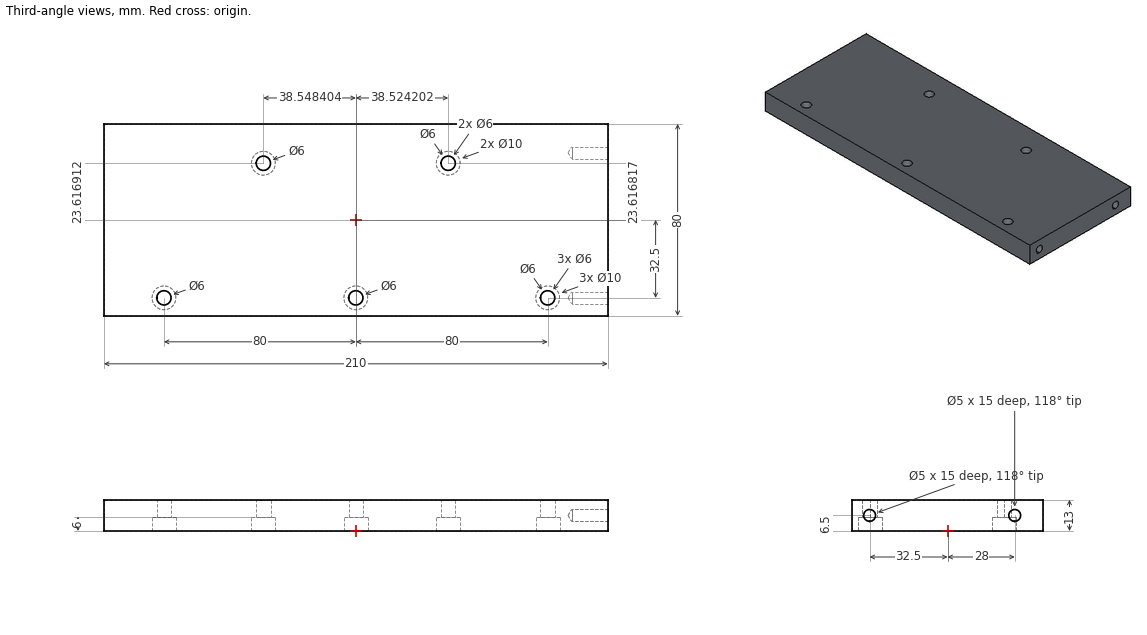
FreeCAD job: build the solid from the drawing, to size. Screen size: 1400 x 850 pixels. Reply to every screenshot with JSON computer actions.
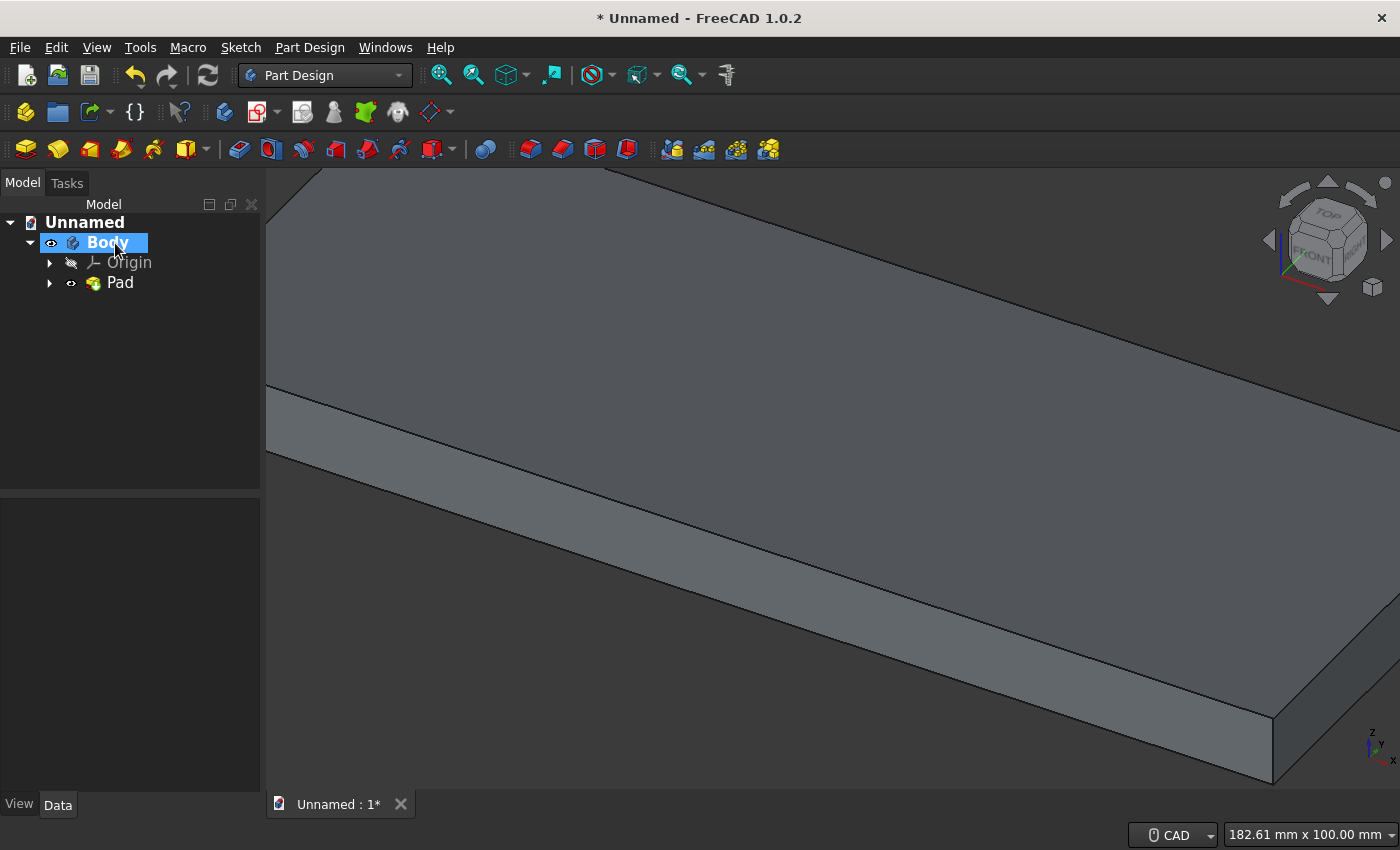
{"action": "key", "text": "v f"}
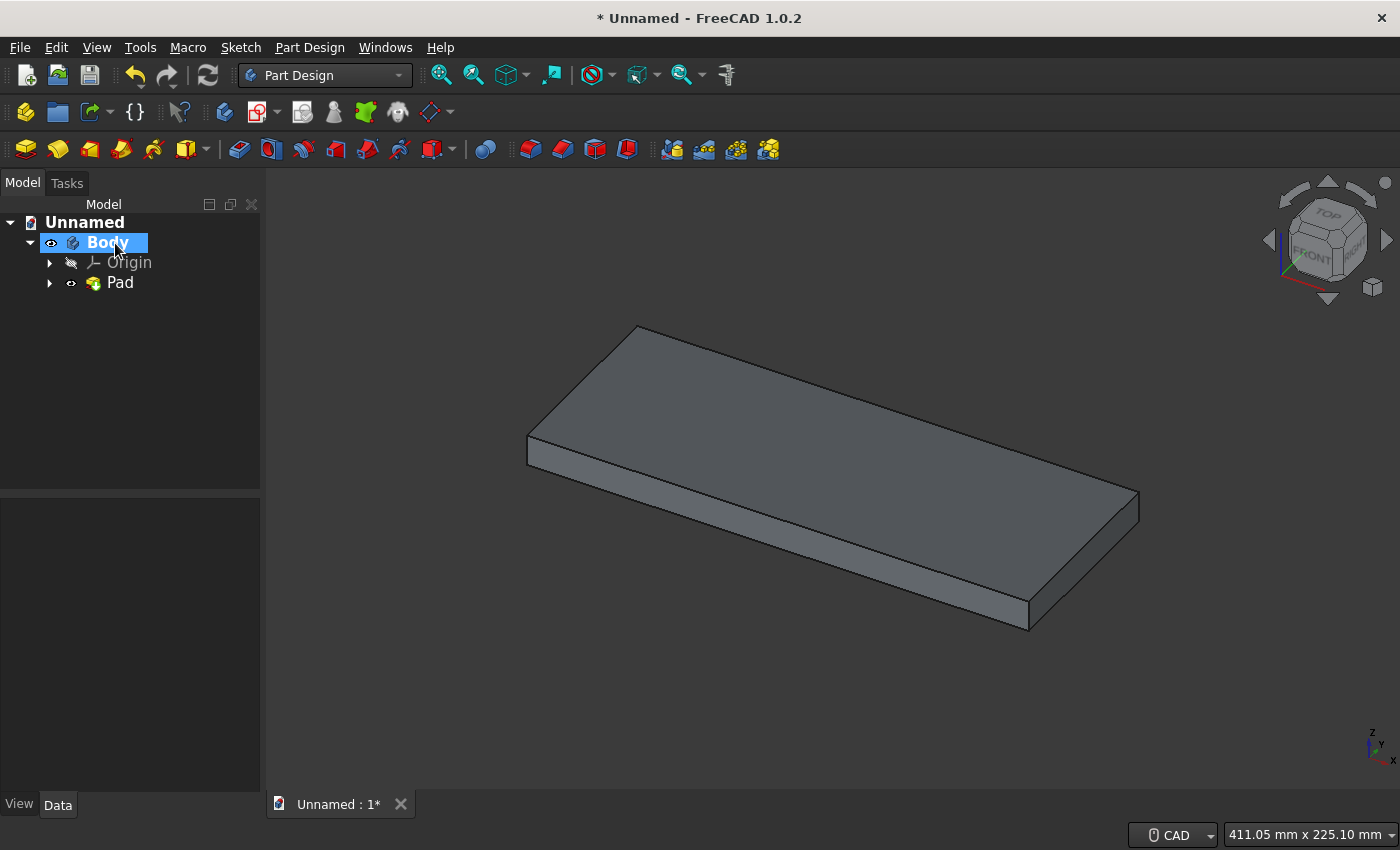
{"action": "left_click", "coordinate": [258, 112]}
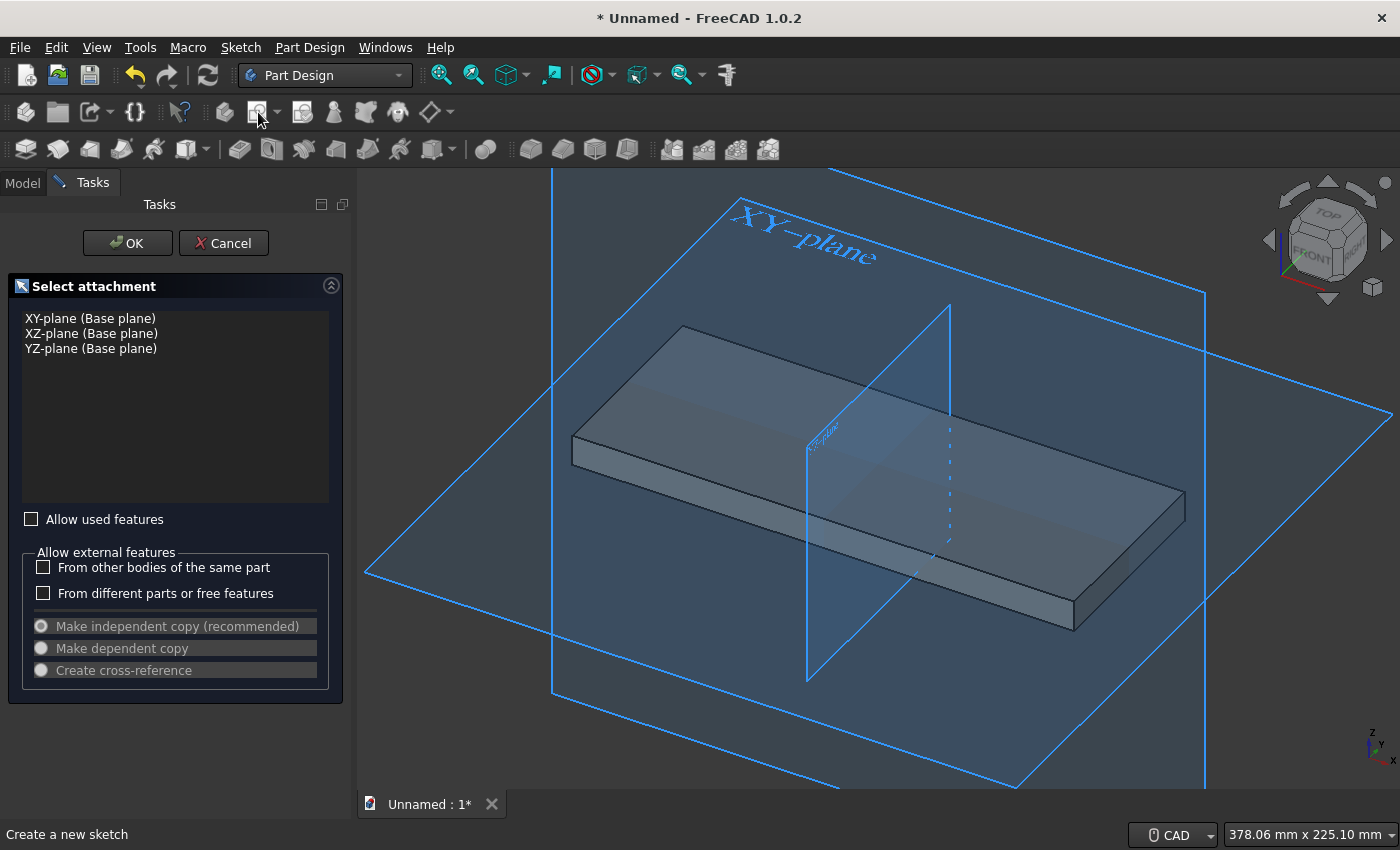
{"action": "left_click", "coordinate": [82, 318]}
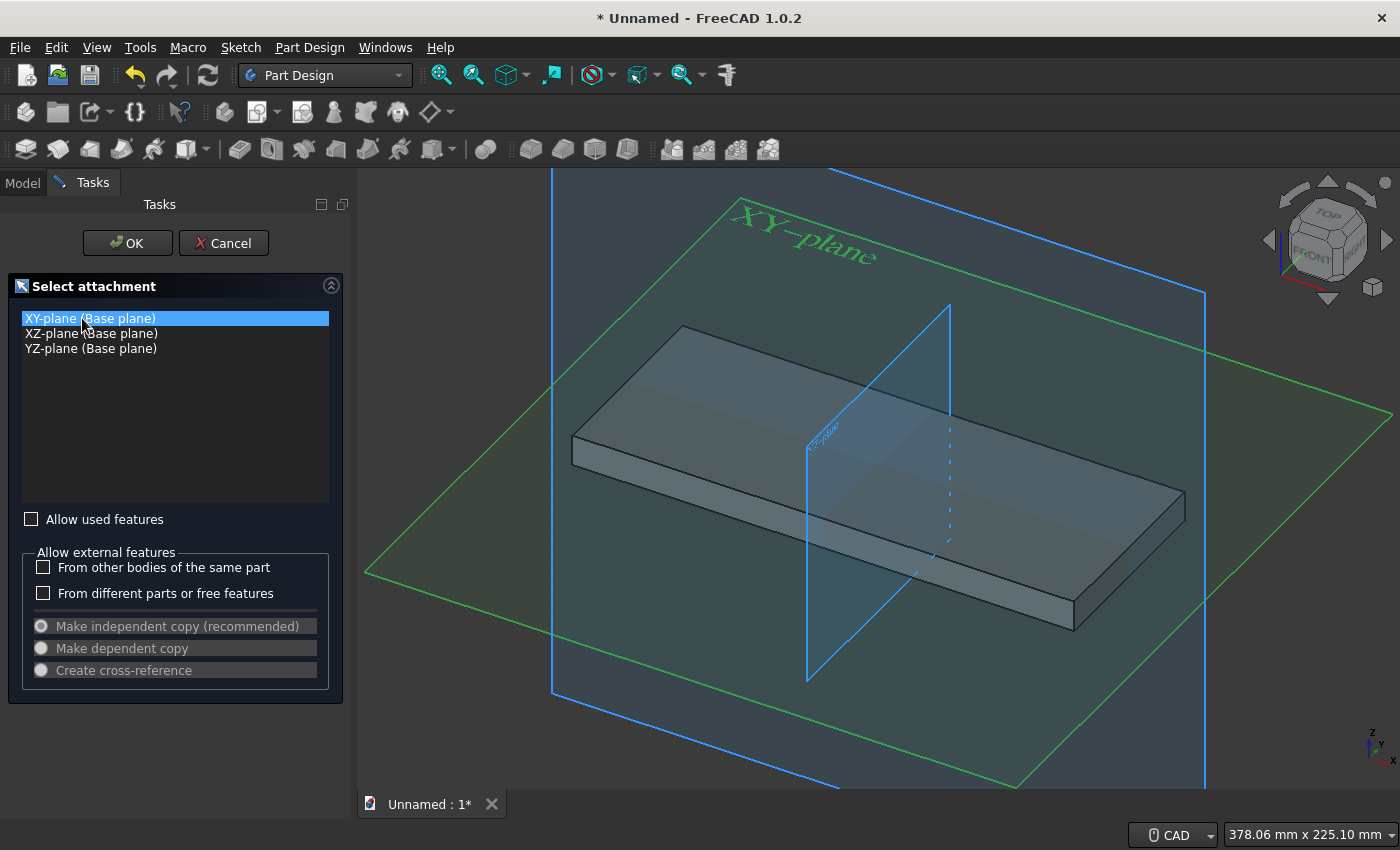
{"action": "left_click", "coordinate": [128, 243]}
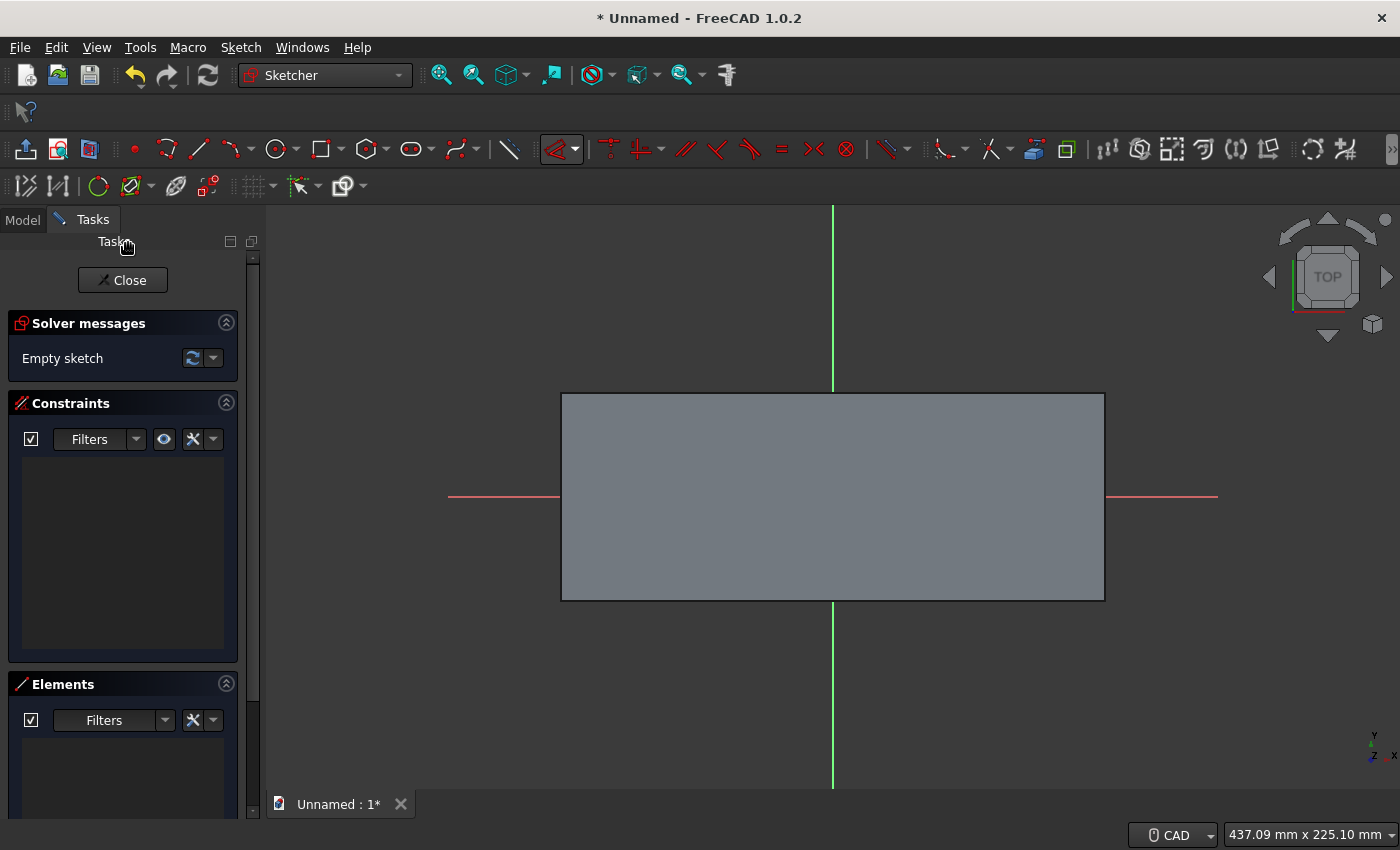
{"action": "key", "text": "q s"}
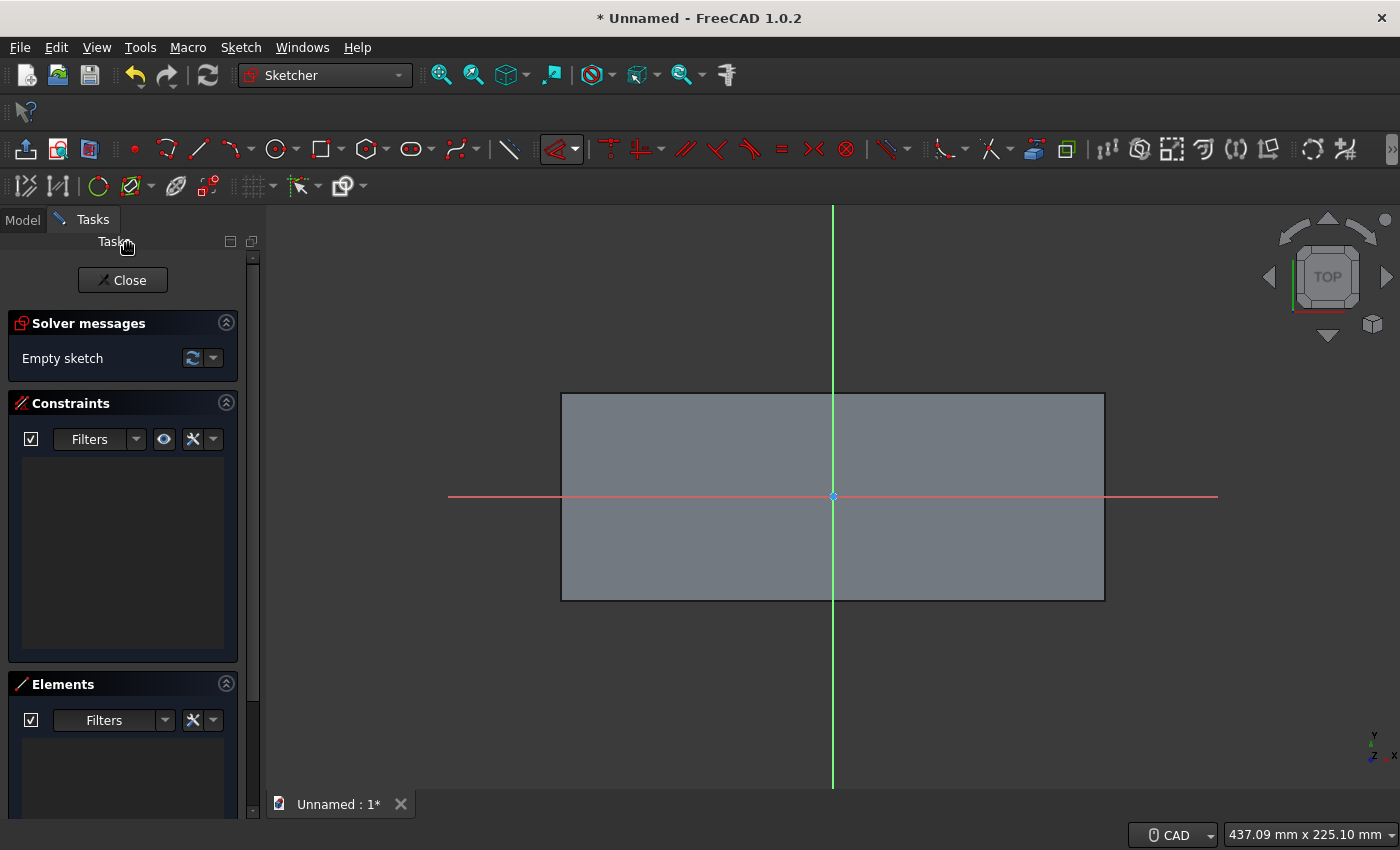
{"action": "scroll", "coordinate": [873, 438], "scroll_direction": "up", "scroll_amount": 5}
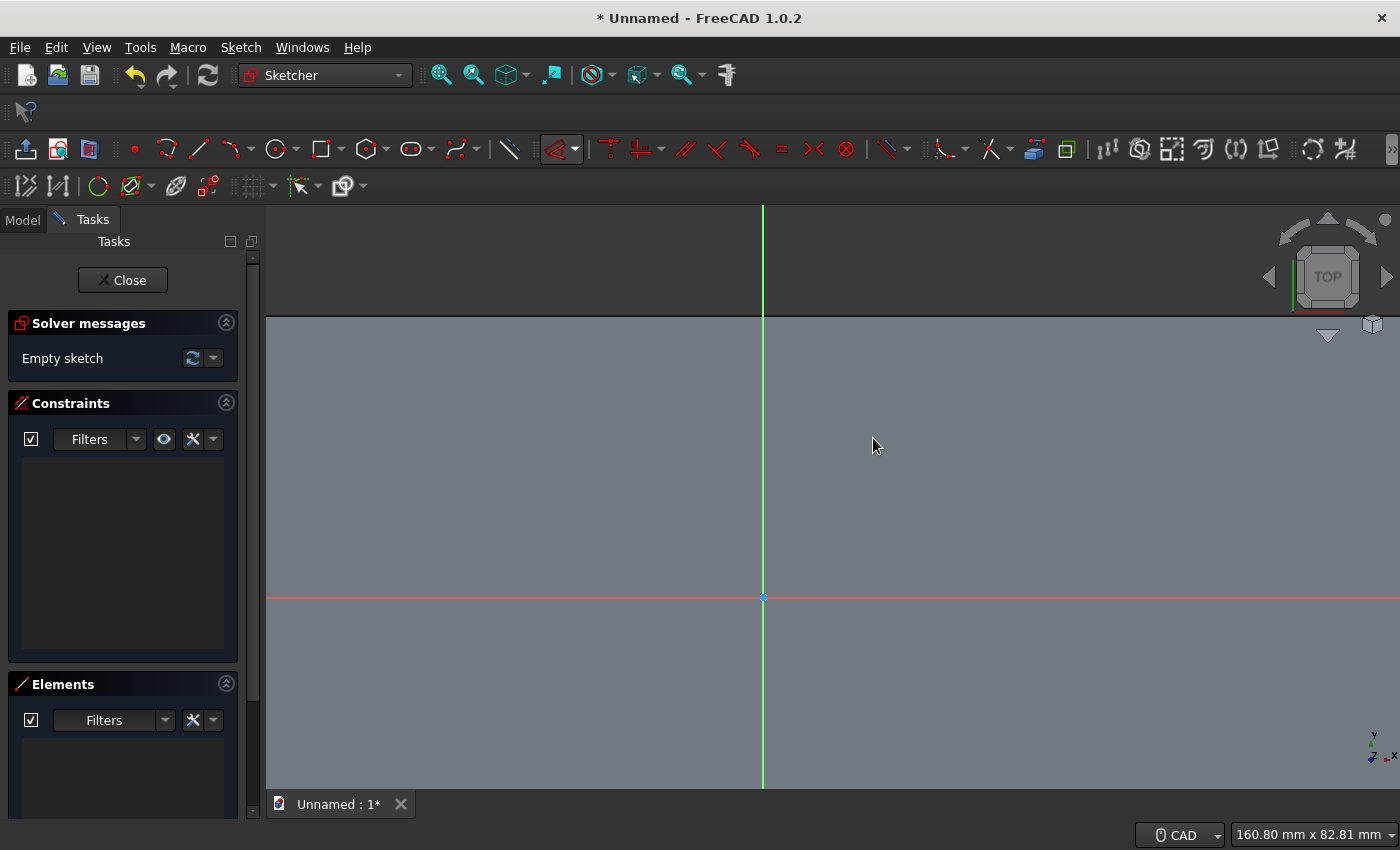
{"action": "left_click", "coordinate": [276, 150]}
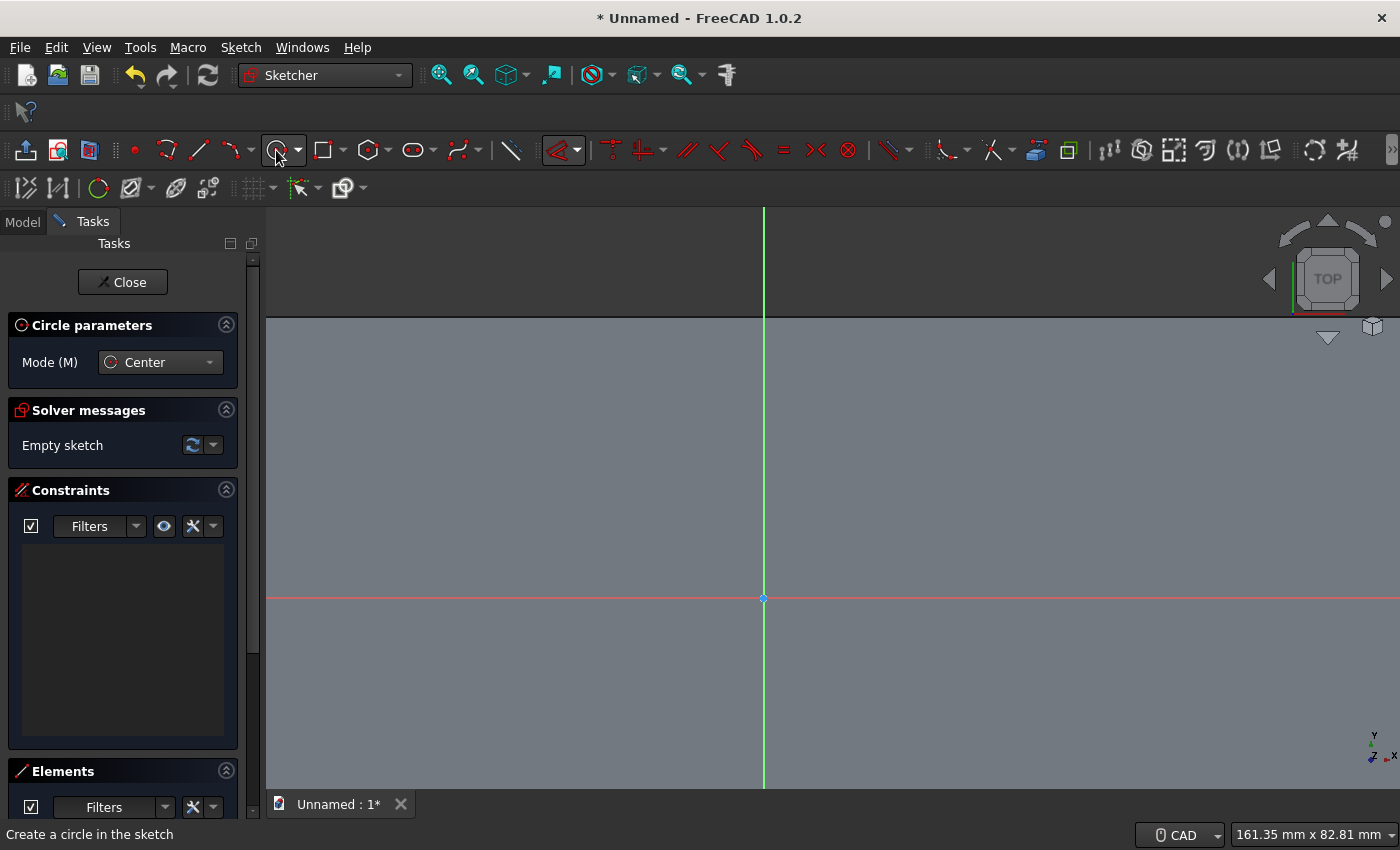
{"action": "left_click", "coordinate": [1034, 432]}
{"action": "left_click", "coordinate": [1059, 408]}